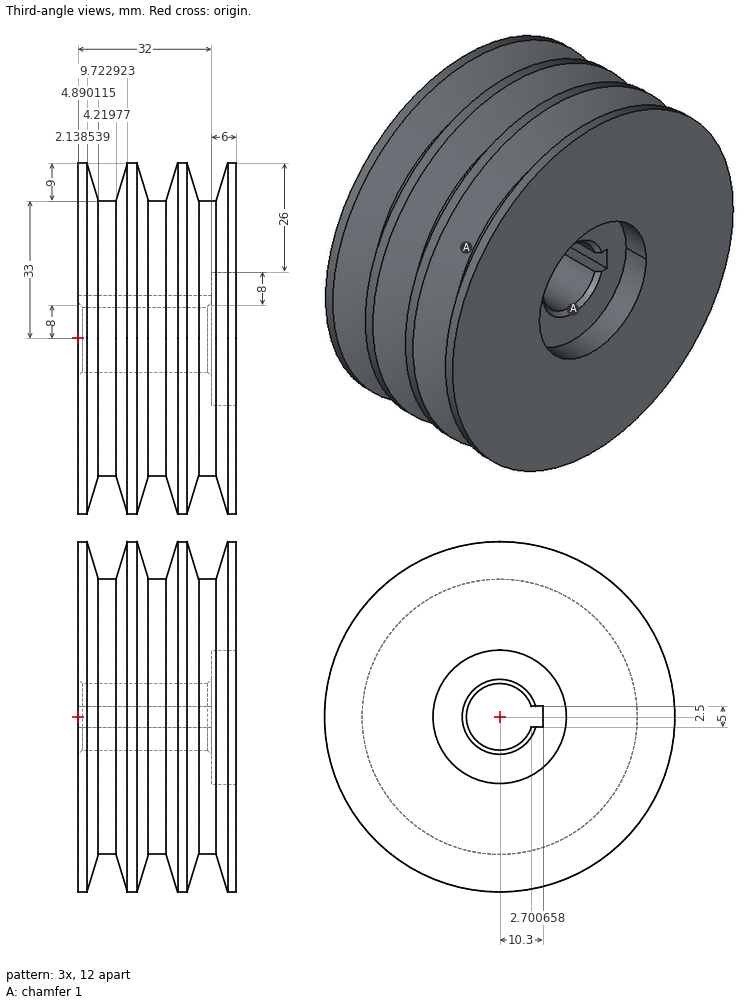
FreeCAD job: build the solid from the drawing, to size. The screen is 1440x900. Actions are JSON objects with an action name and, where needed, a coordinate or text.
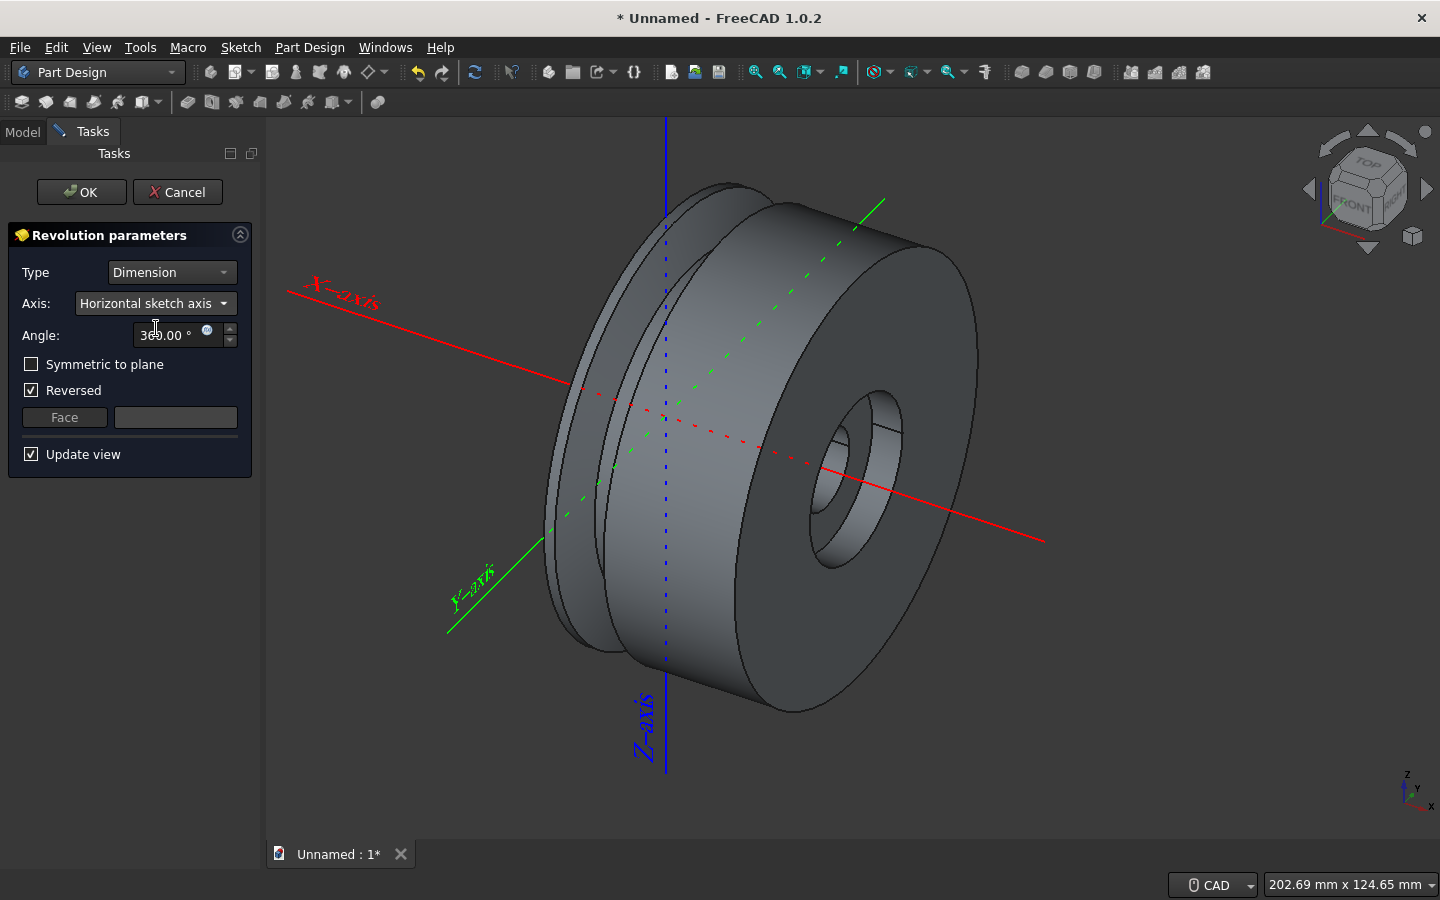
{"action": "left_click", "coordinate": [82, 192]}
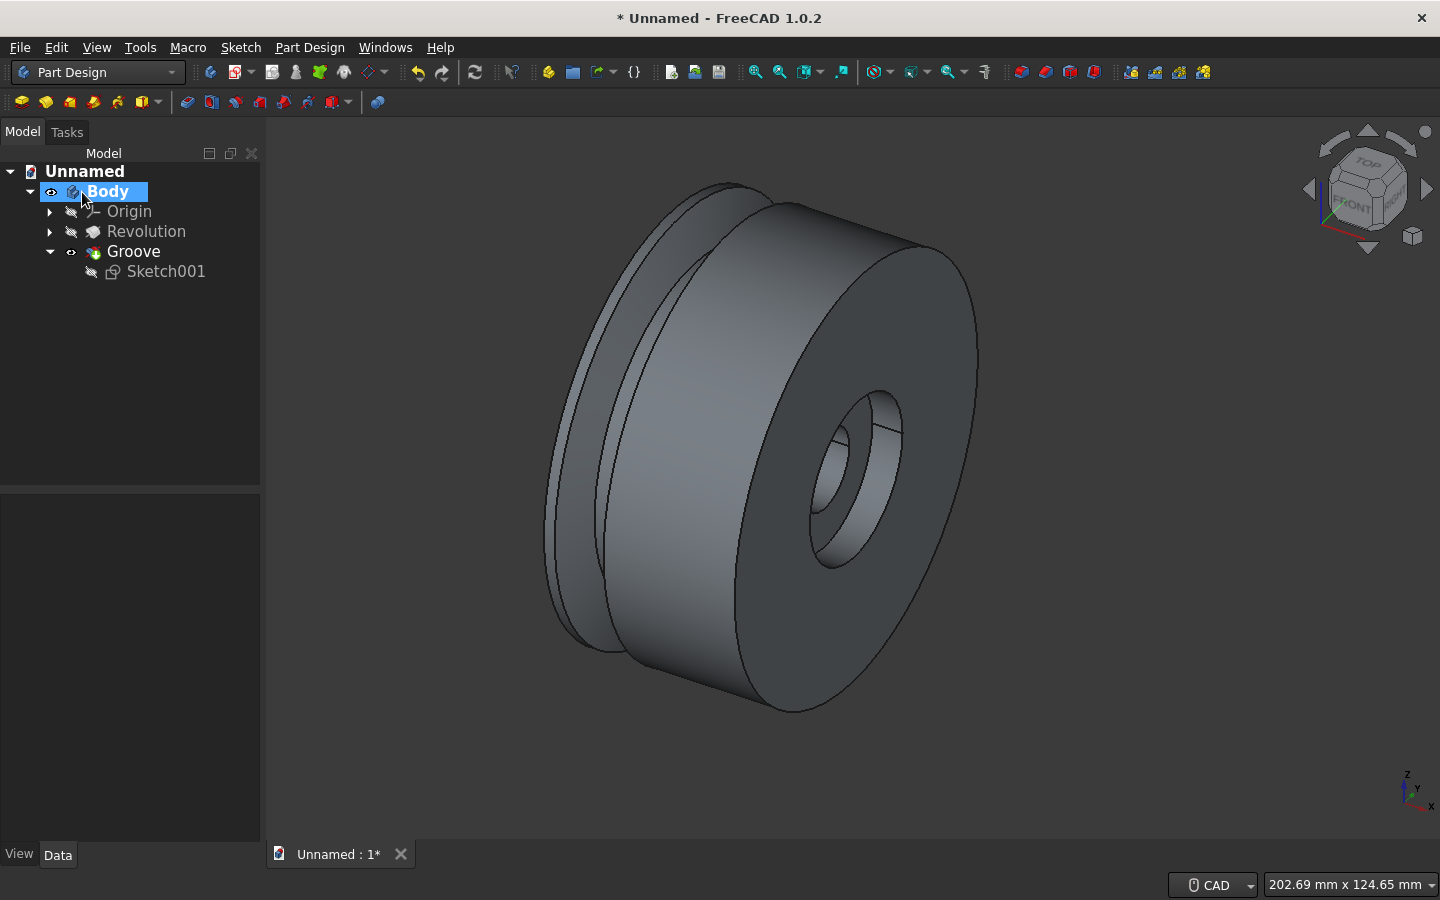
{"action": "key", "text": "v f"}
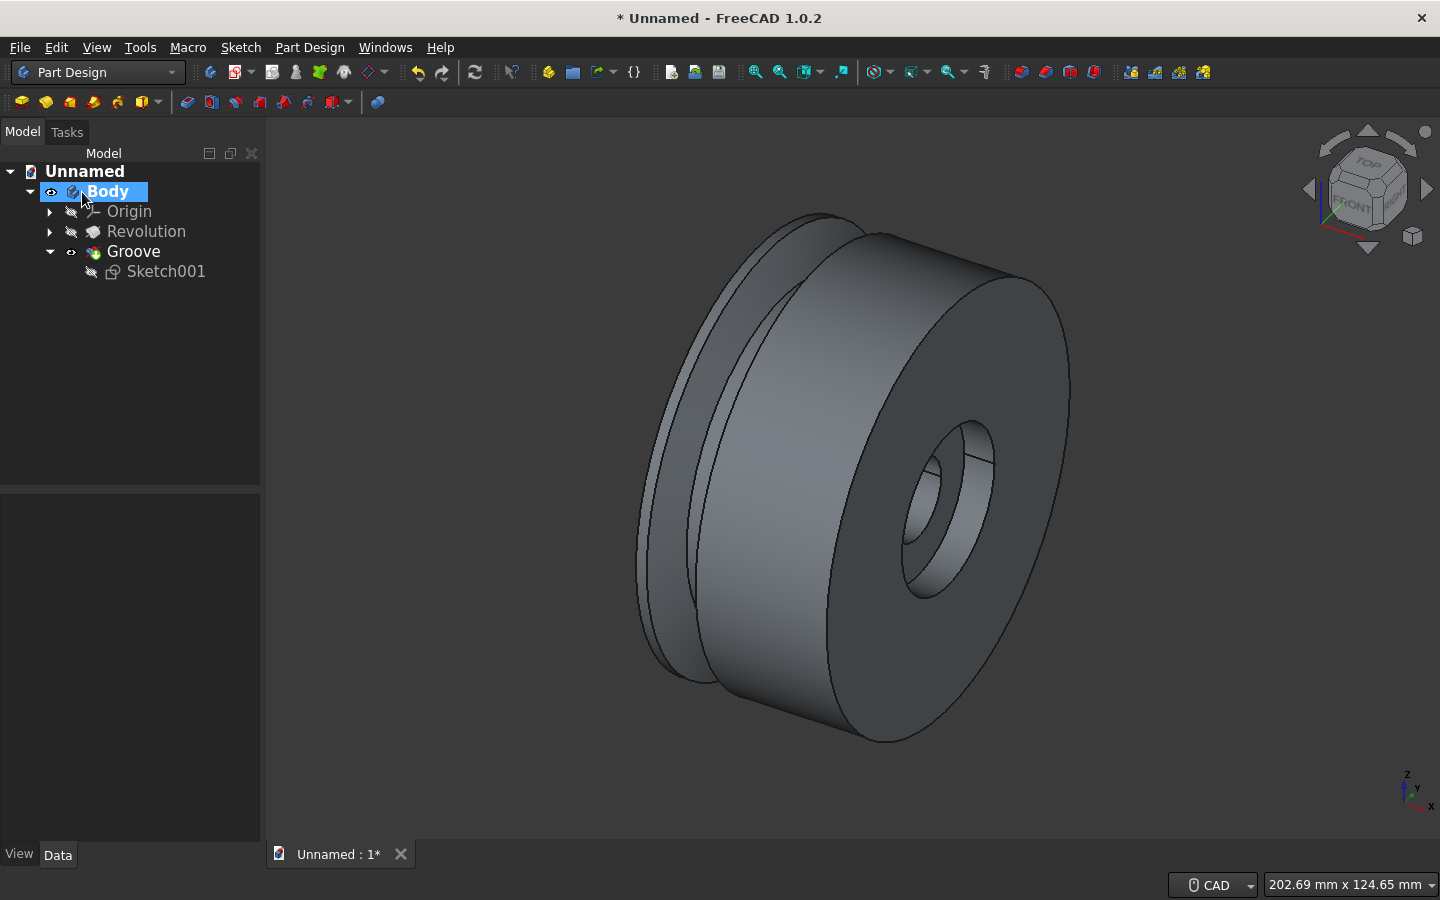
{"action": "left_click", "coordinate": [116, 252]}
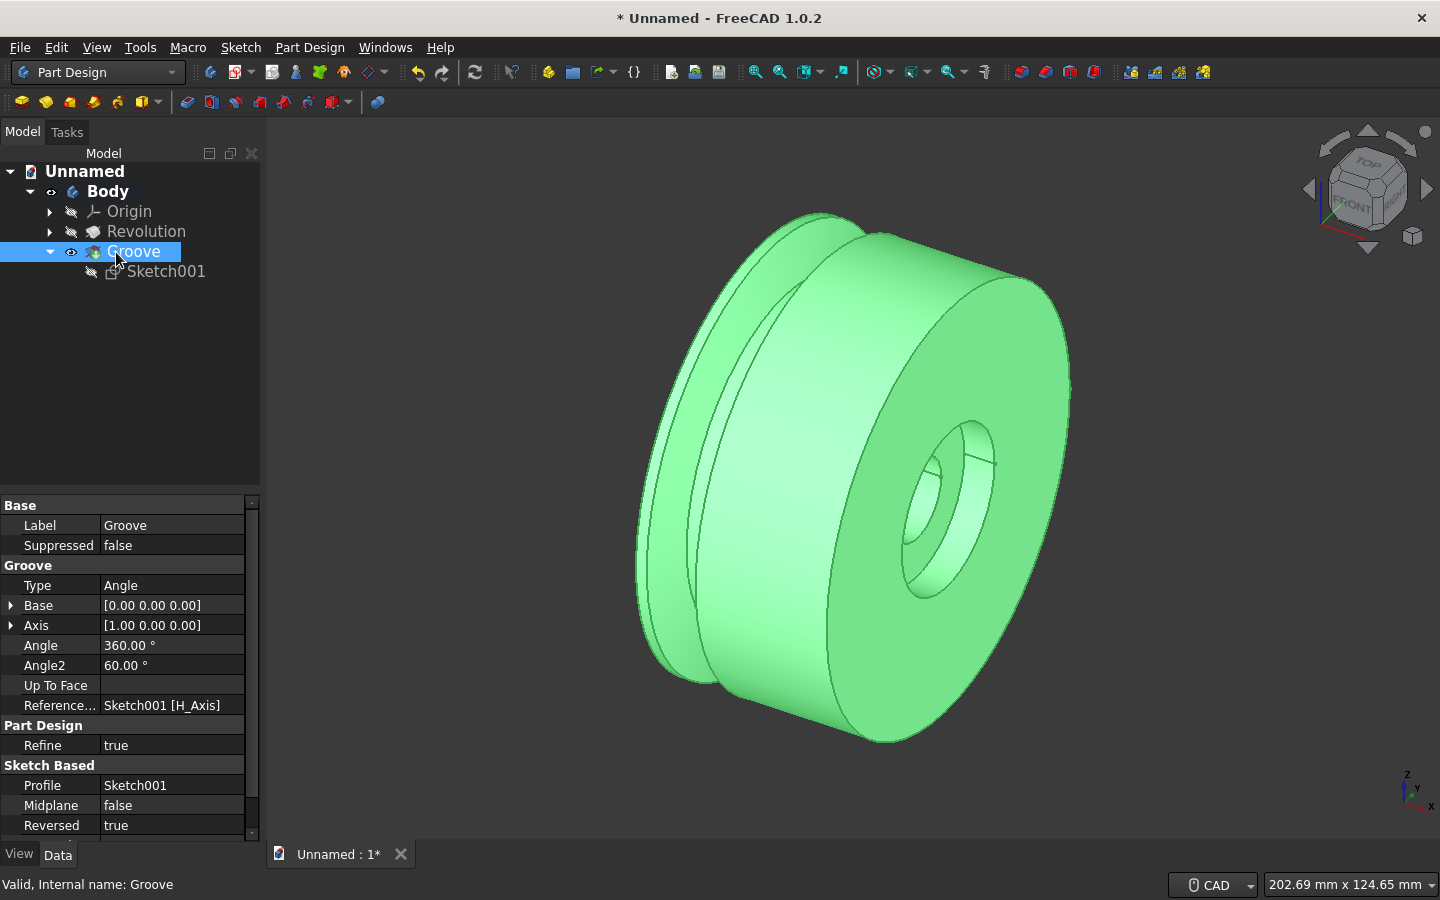
{"action": "left_click", "coordinate": [1156, 72]}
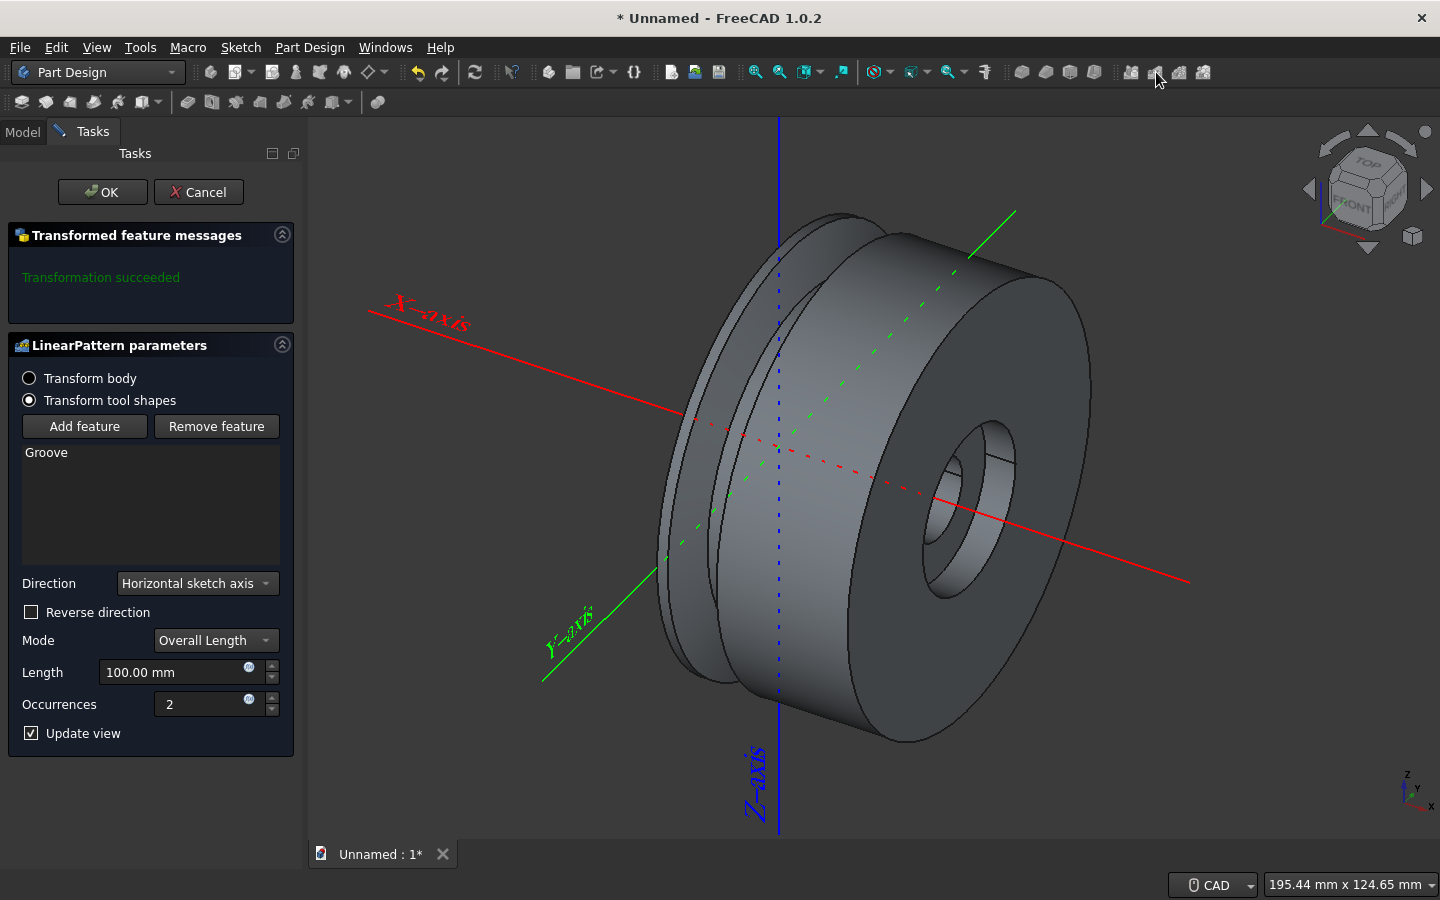
{"action": "left_click", "coordinate": [198, 584]}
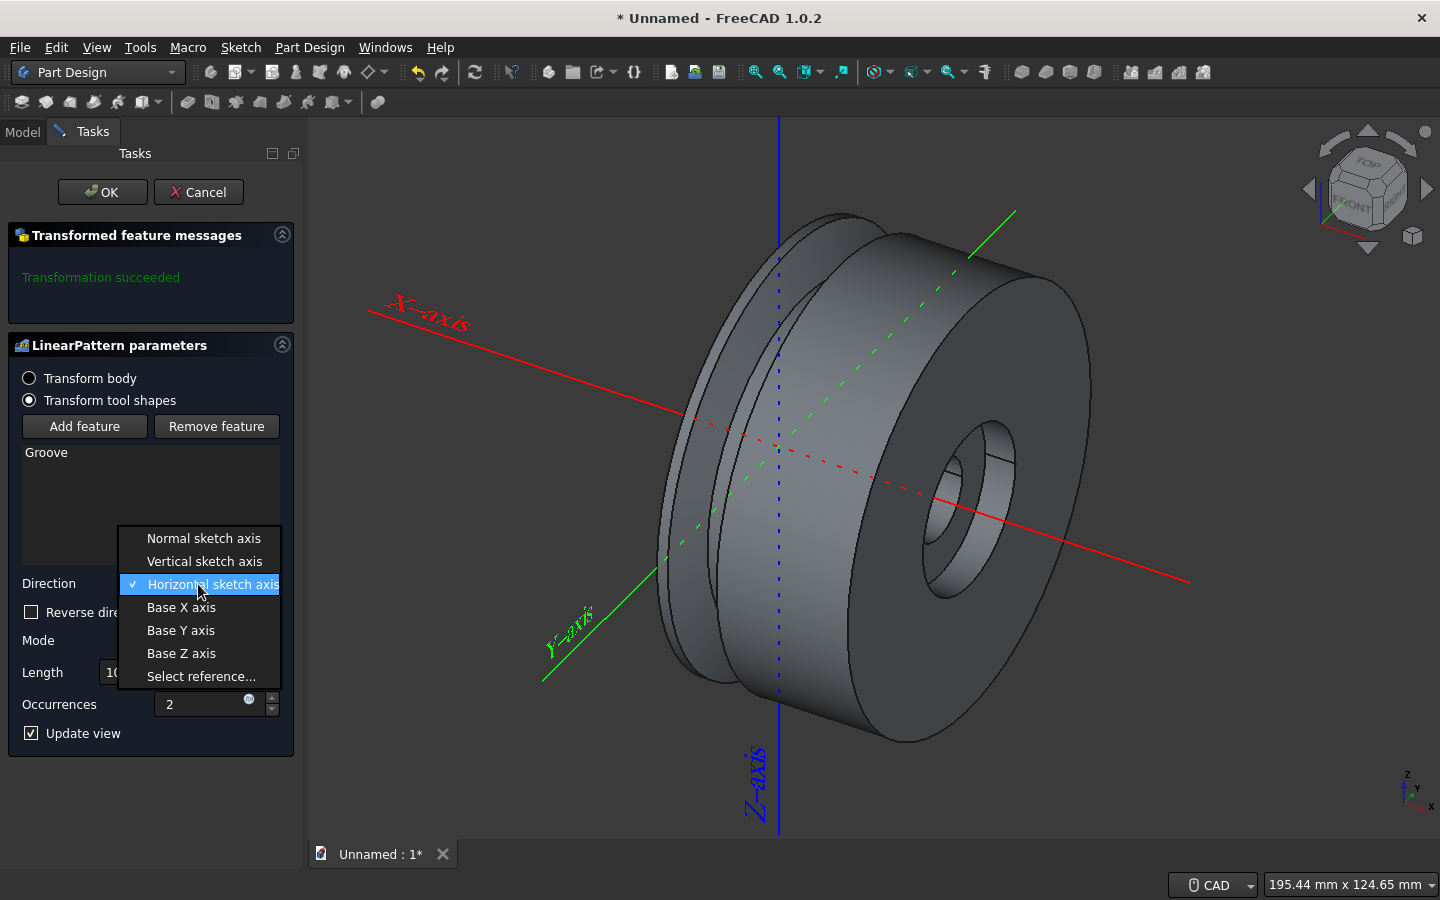
{"action": "left_click", "coordinate": [198, 608]}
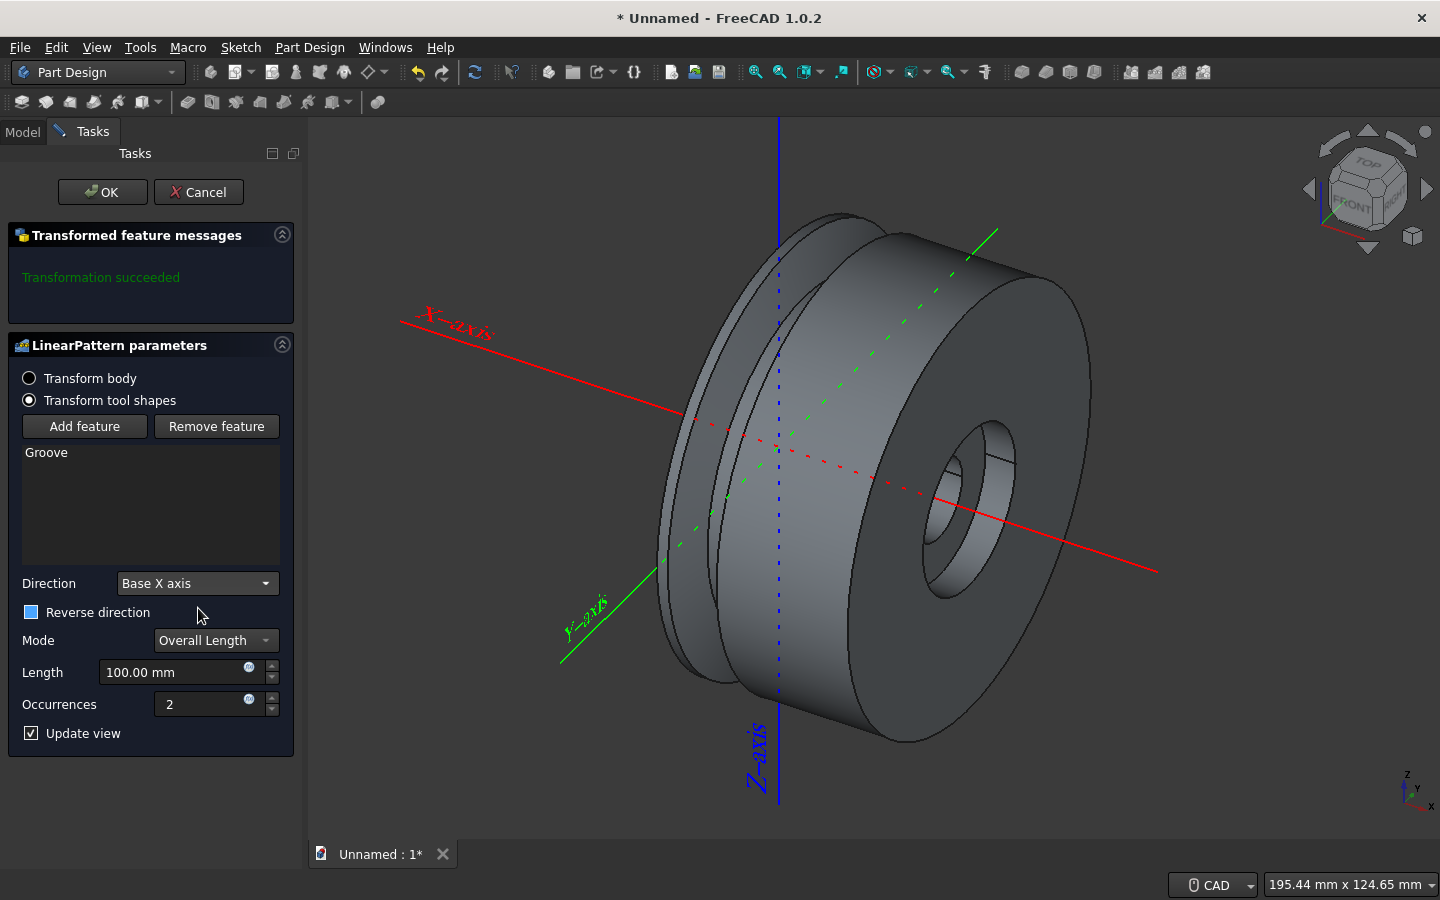
{"action": "left_click", "coordinate": [217, 640]}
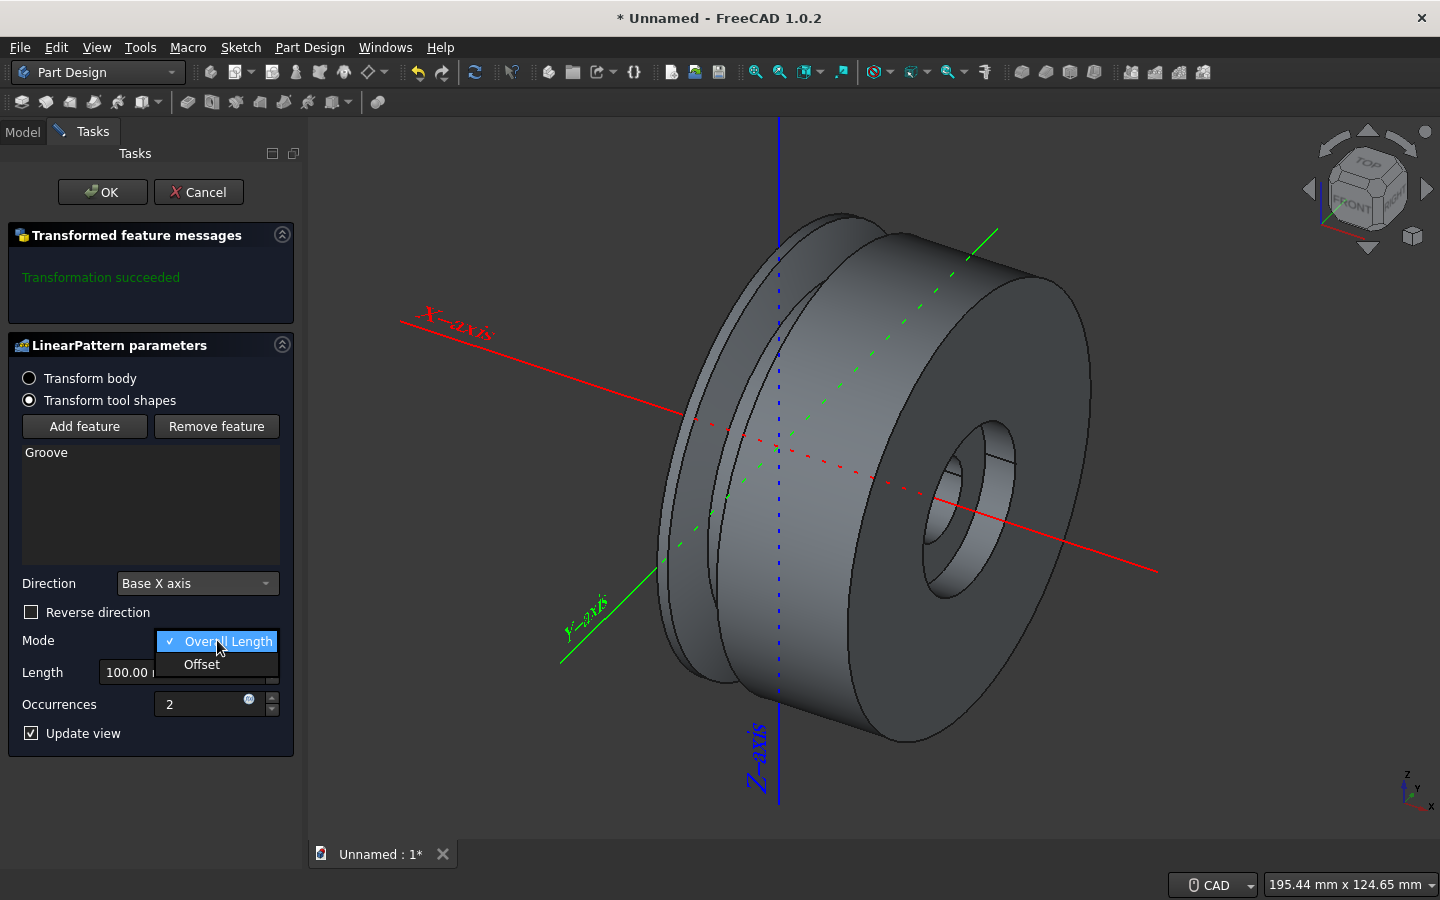
{"action": "left_click", "coordinate": [216, 664]}